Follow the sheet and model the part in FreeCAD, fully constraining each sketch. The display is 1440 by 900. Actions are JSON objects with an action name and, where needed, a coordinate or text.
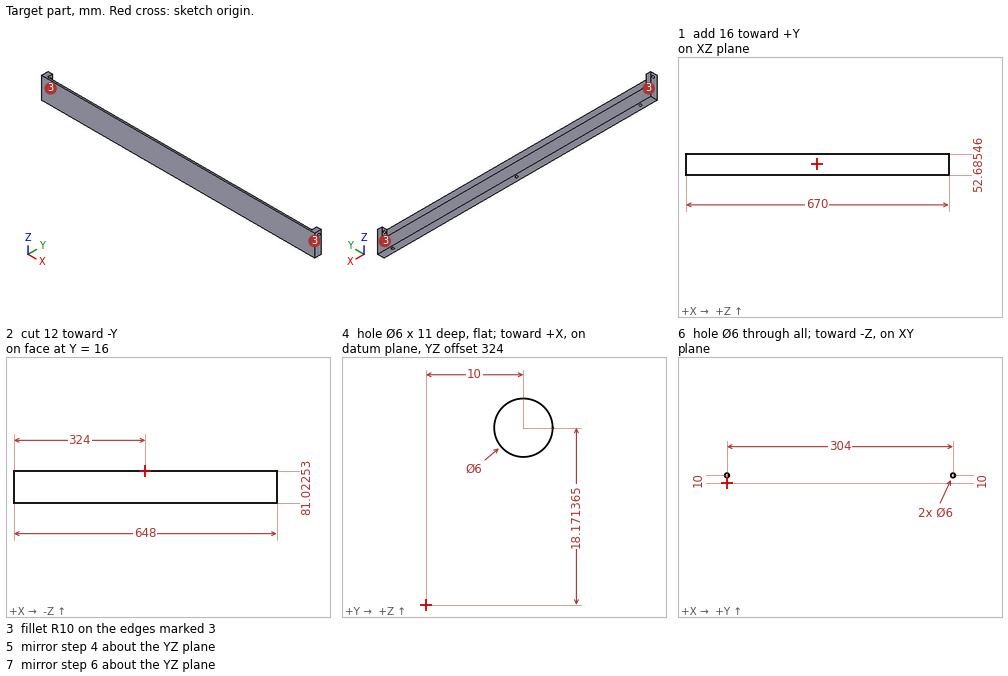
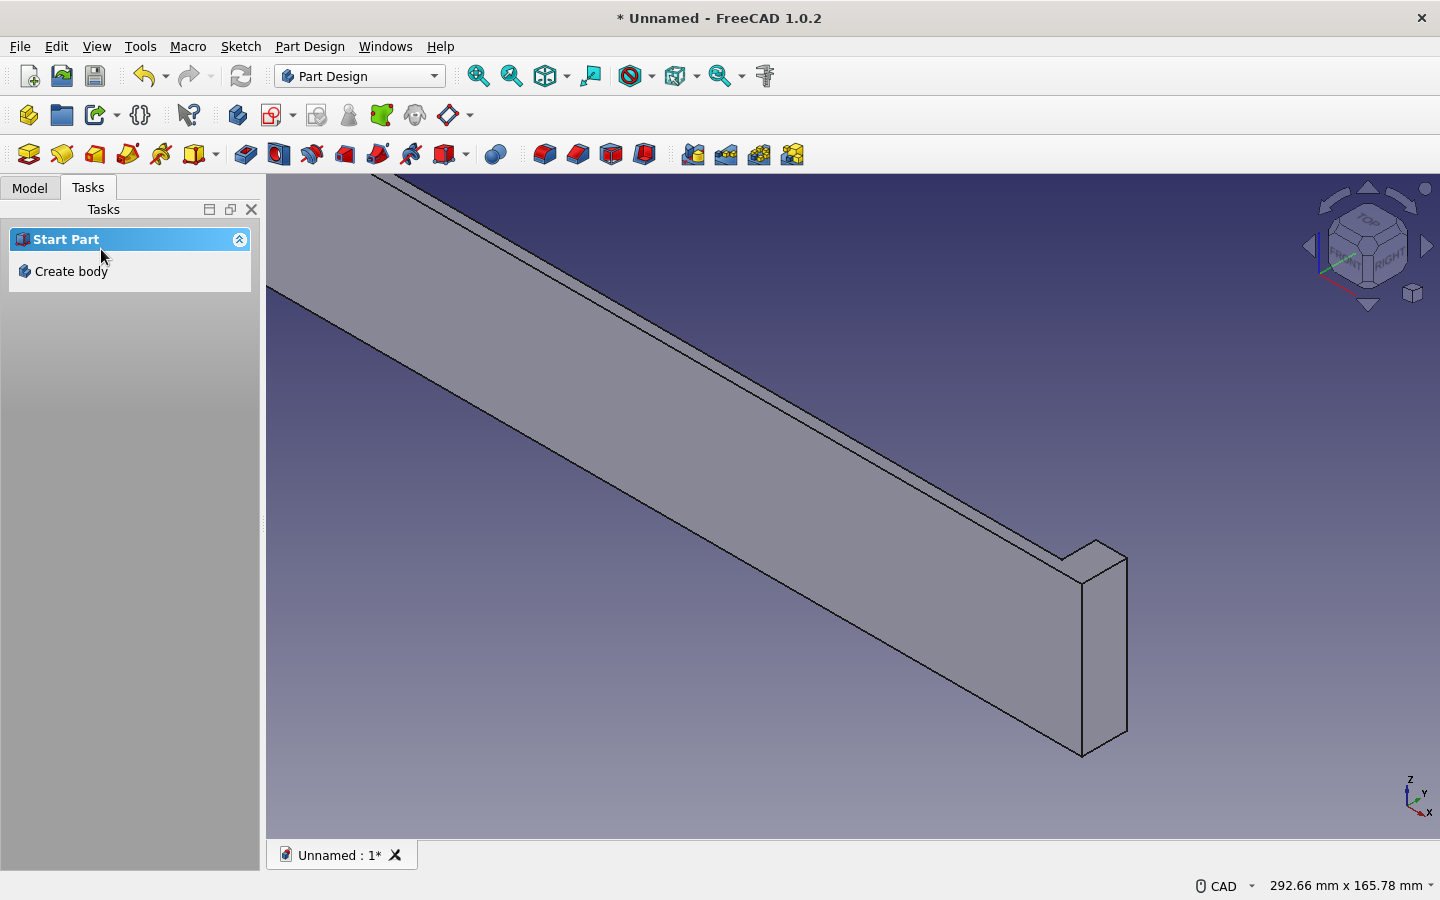
{"action": "left_click", "coordinate": [479, 76]}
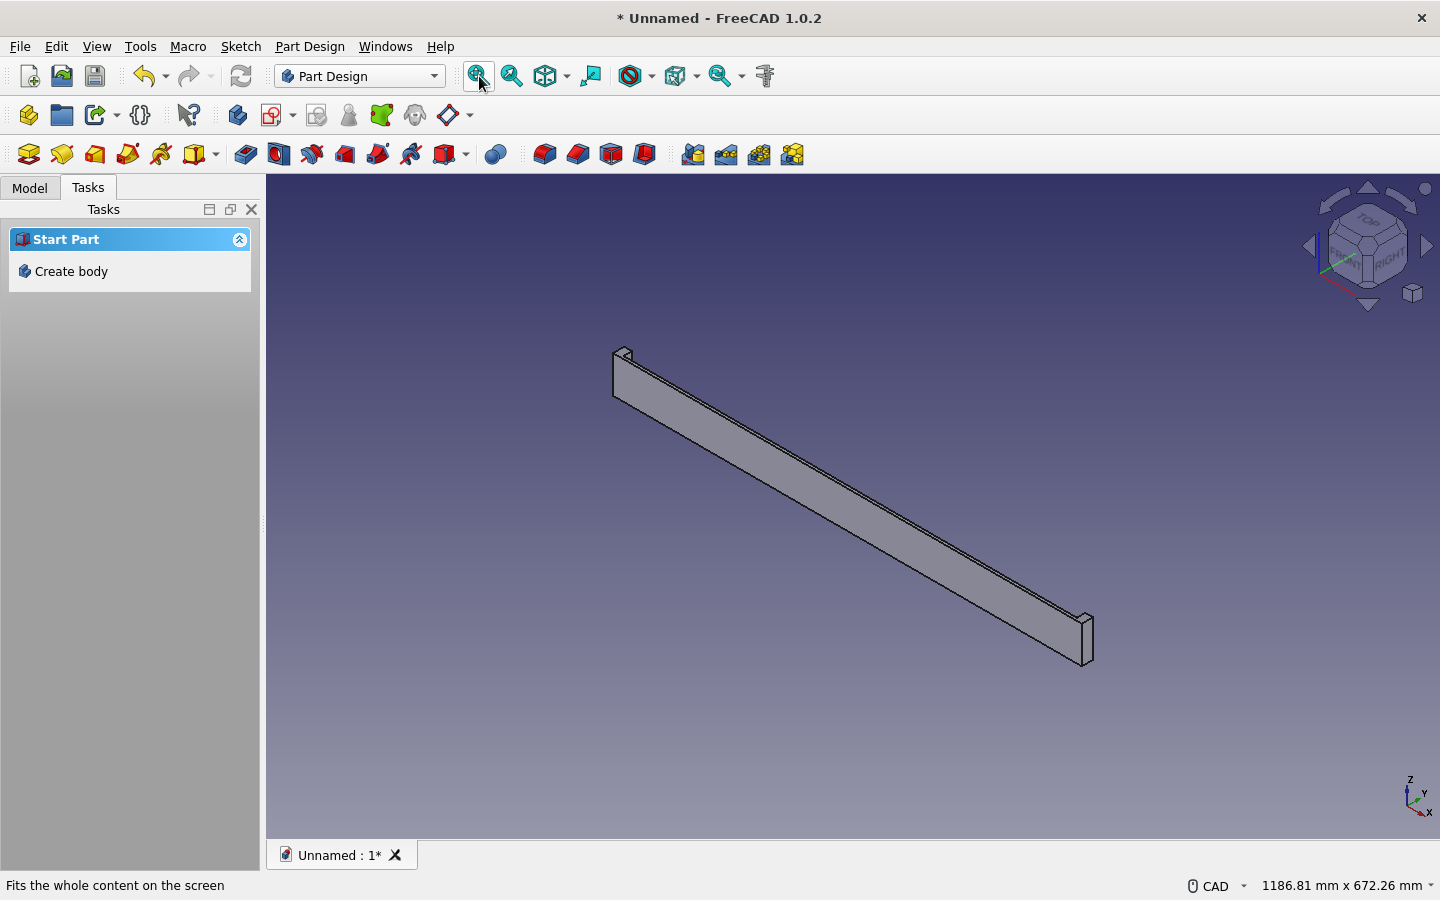
{"action": "left_click", "coordinate": [30, 188]}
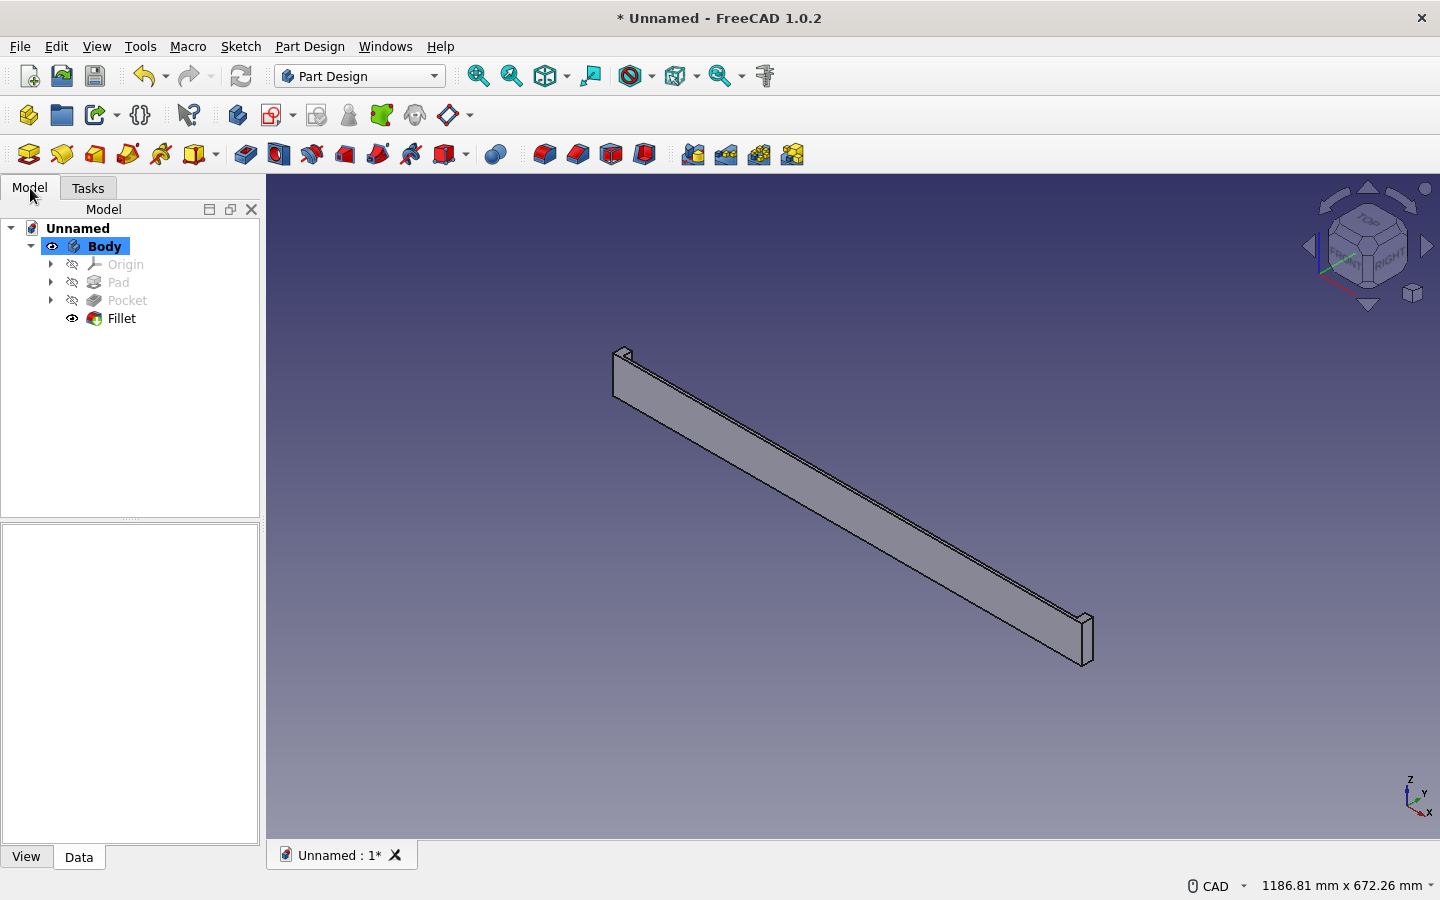
{"action": "left_click", "coordinate": [51, 264]}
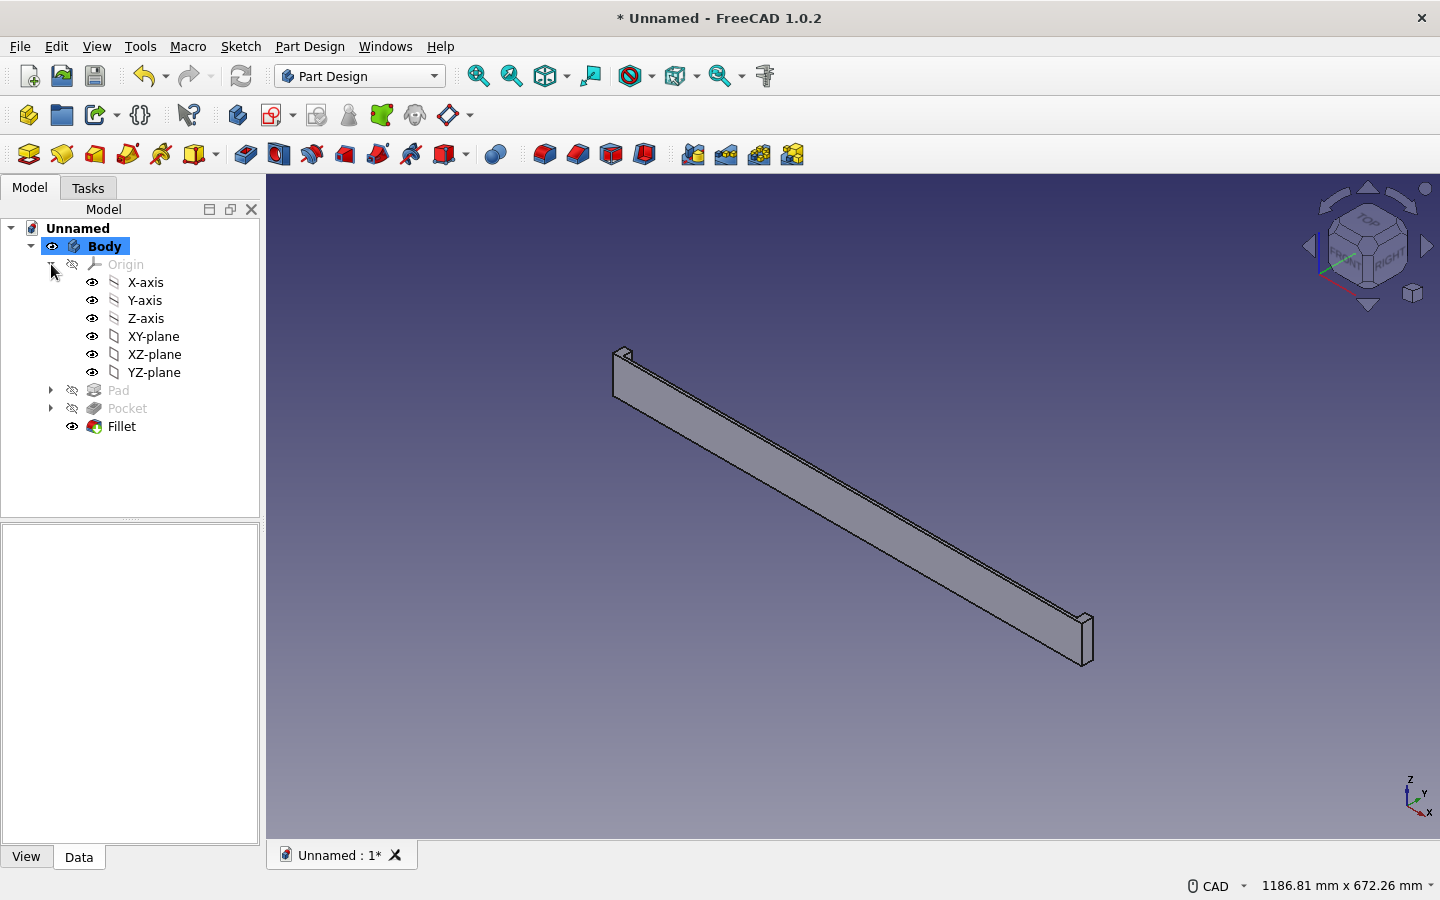
{"action": "left_click", "coordinate": [137, 372]}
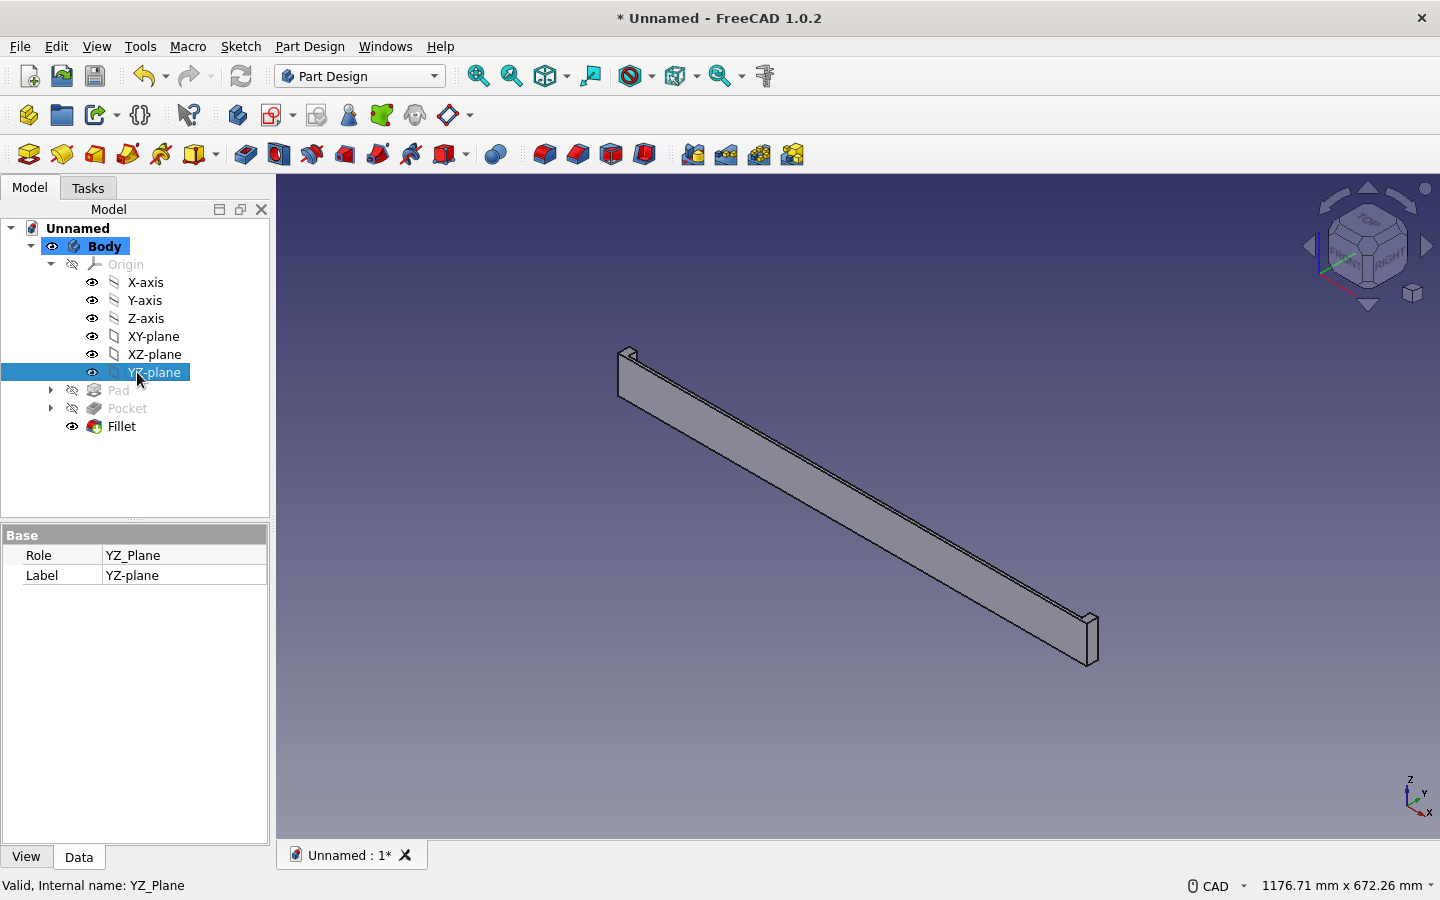
{"action": "left_click", "coordinate": [448, 116]}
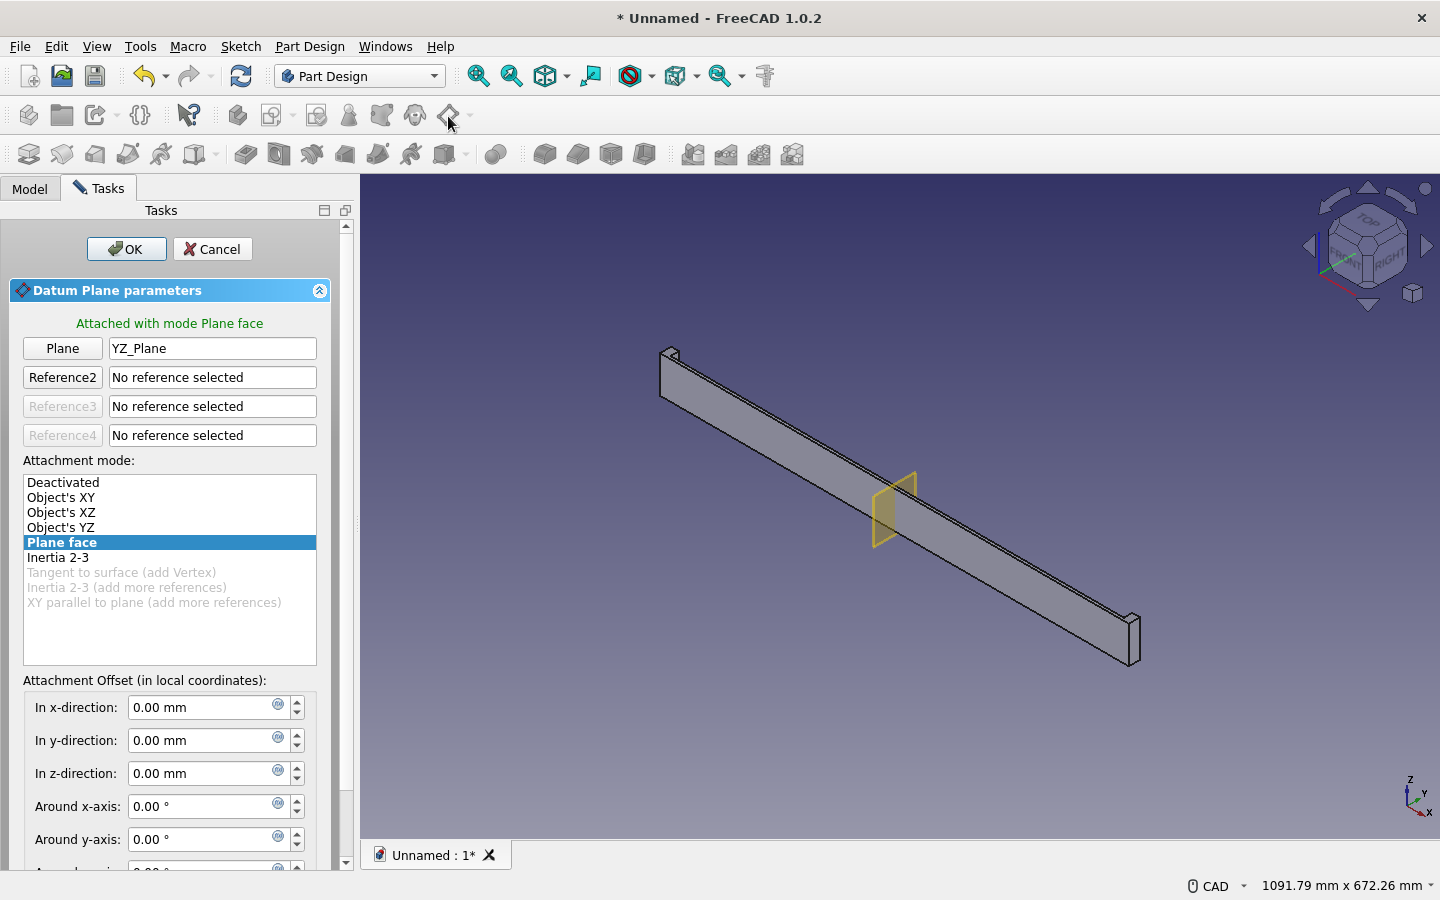
{"action": "triple_click", "coordinate": [210, 774]}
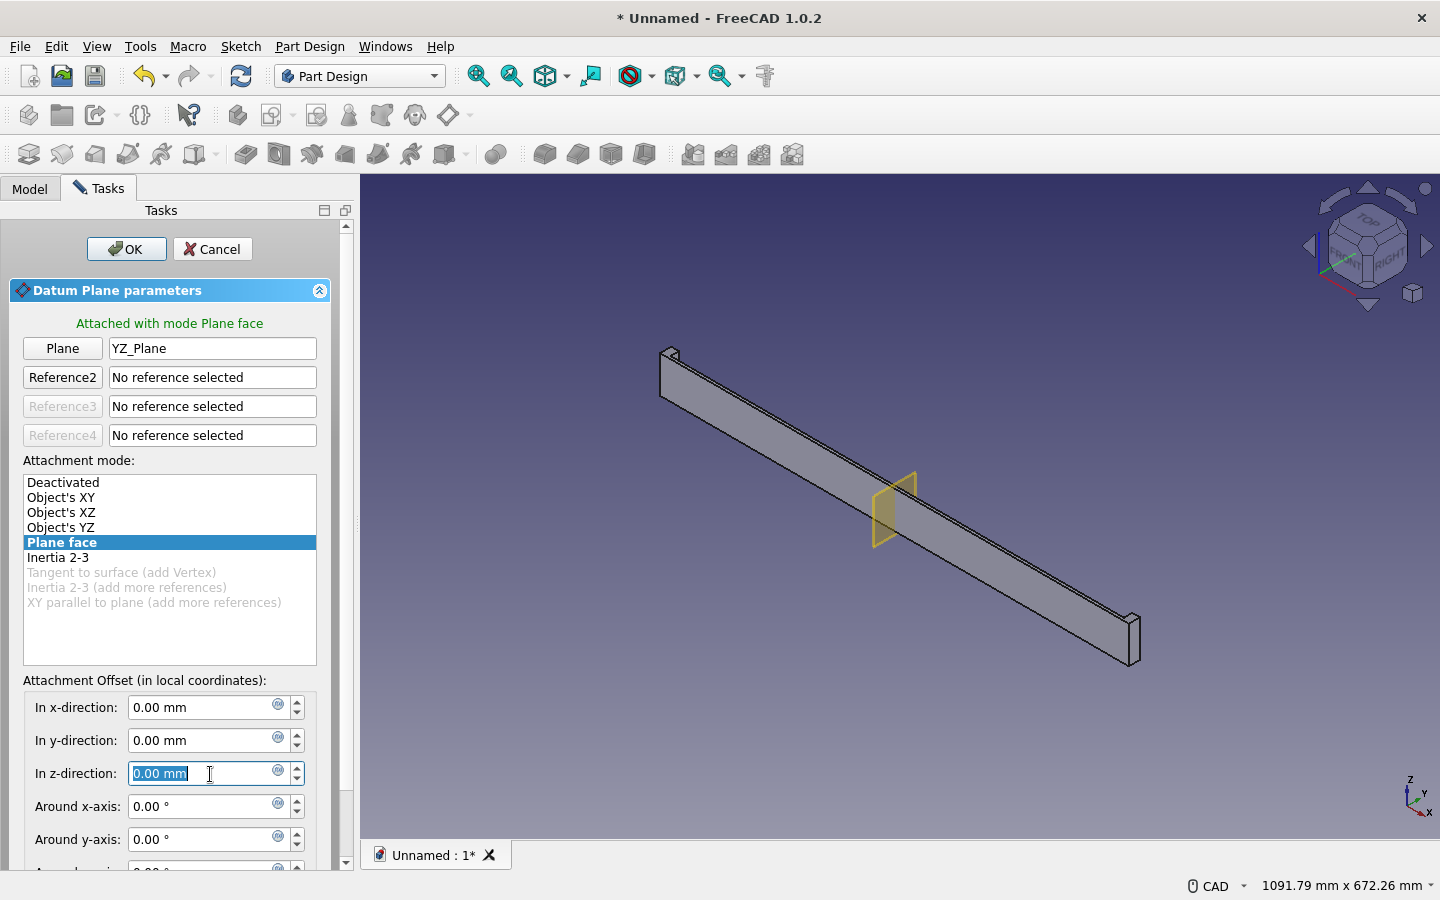
{"action": "type", "text": "324"}
{"action": "key", "text": "Tab"}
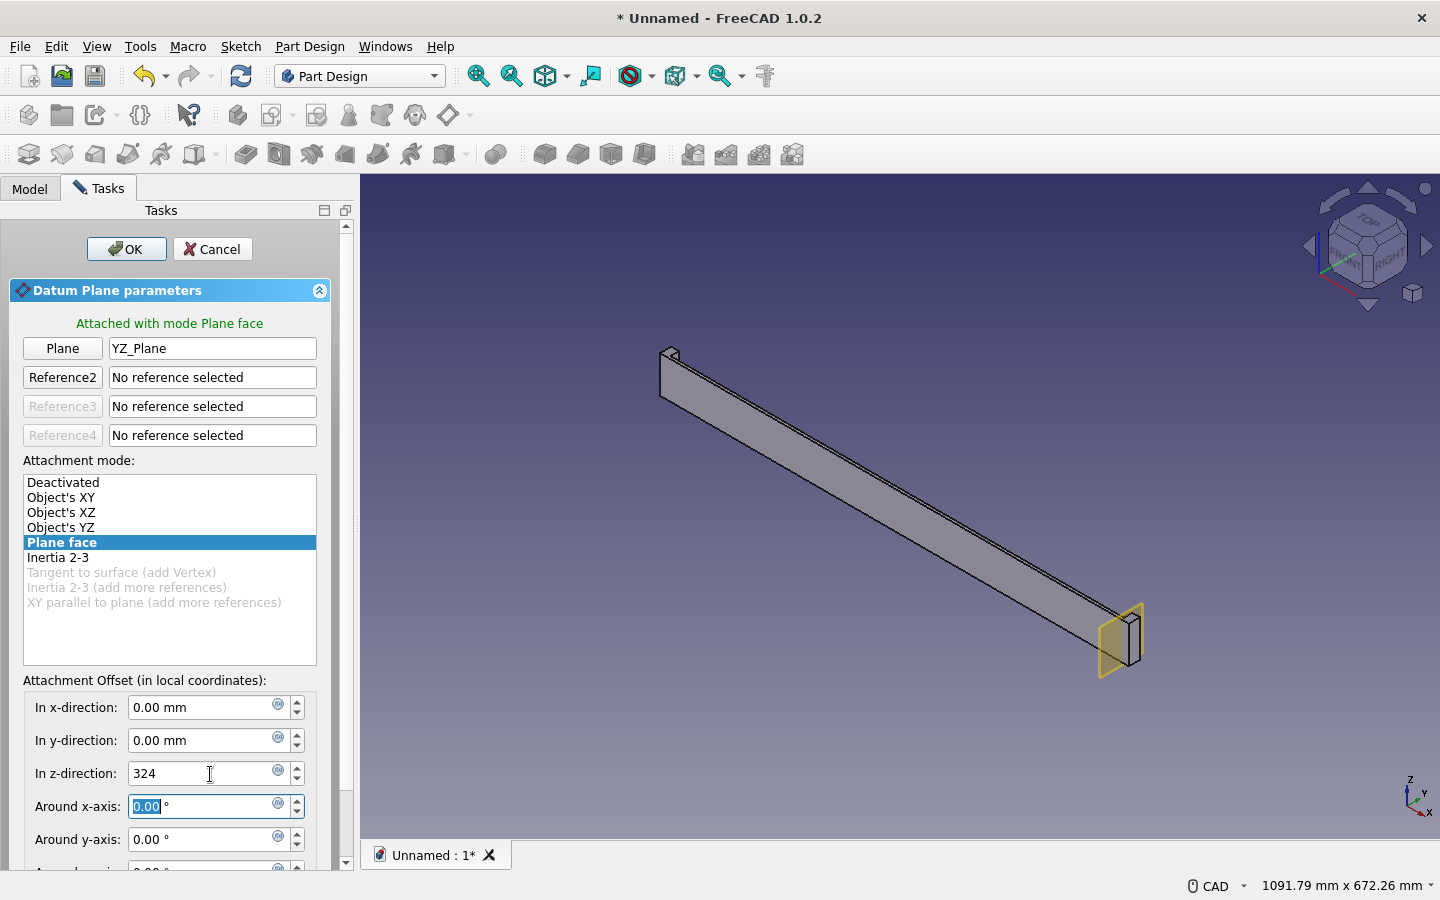
{"action": "left_click", "coordinate": [127, 249]}